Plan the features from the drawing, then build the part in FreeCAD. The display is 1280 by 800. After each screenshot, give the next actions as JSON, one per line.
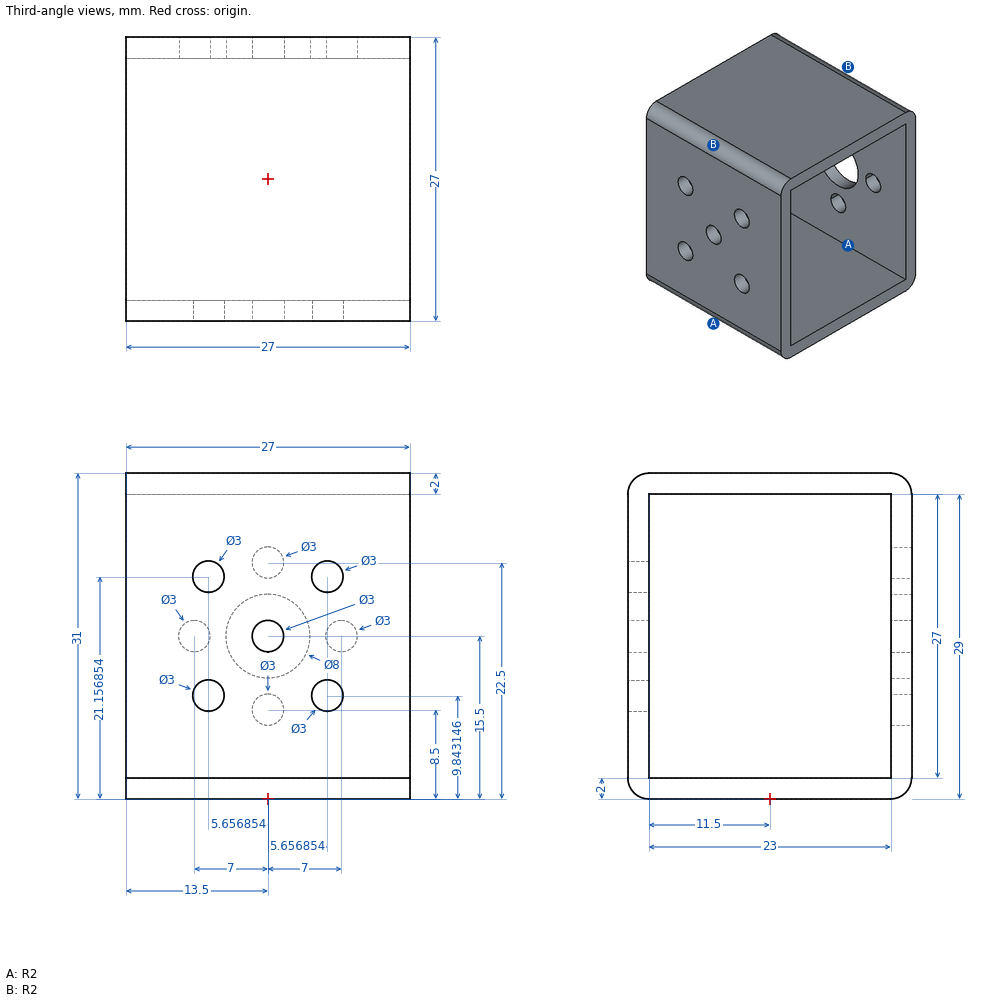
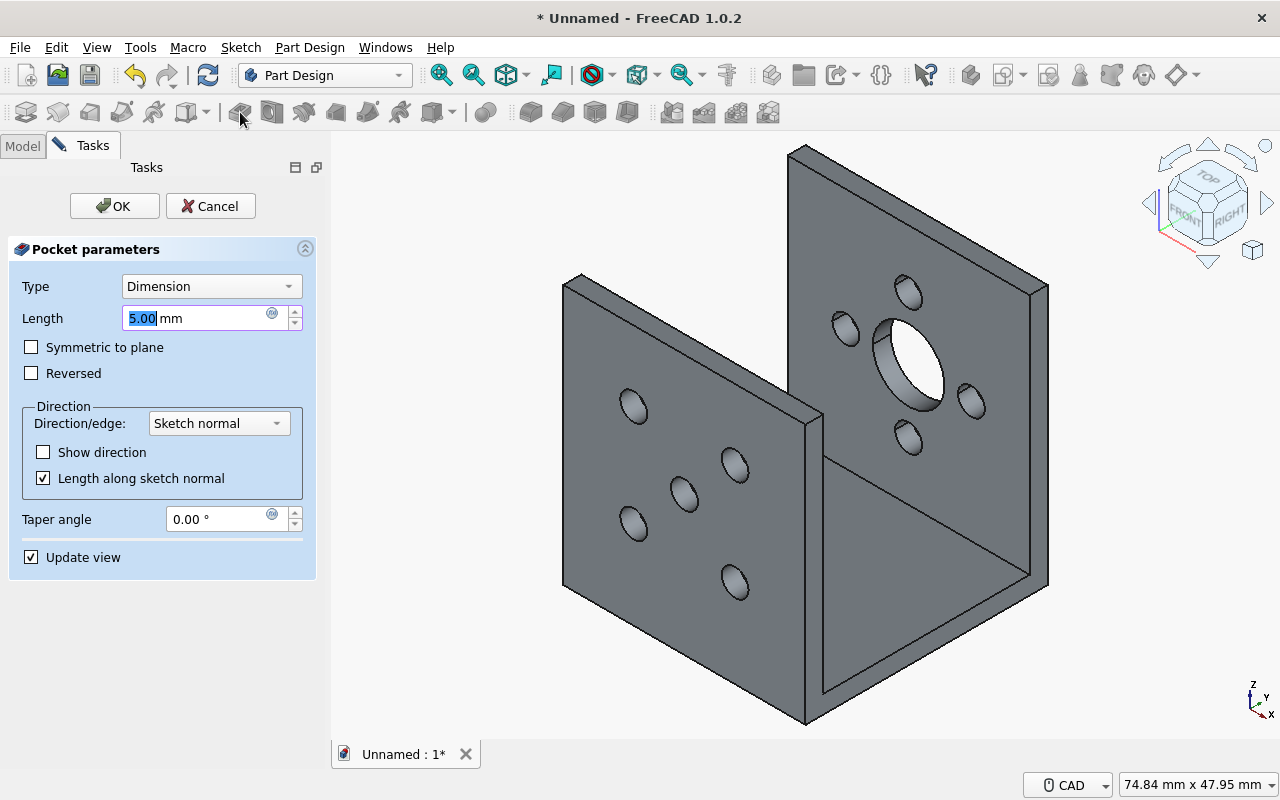
{"action": "left_click", "coordinate": [212, 286]}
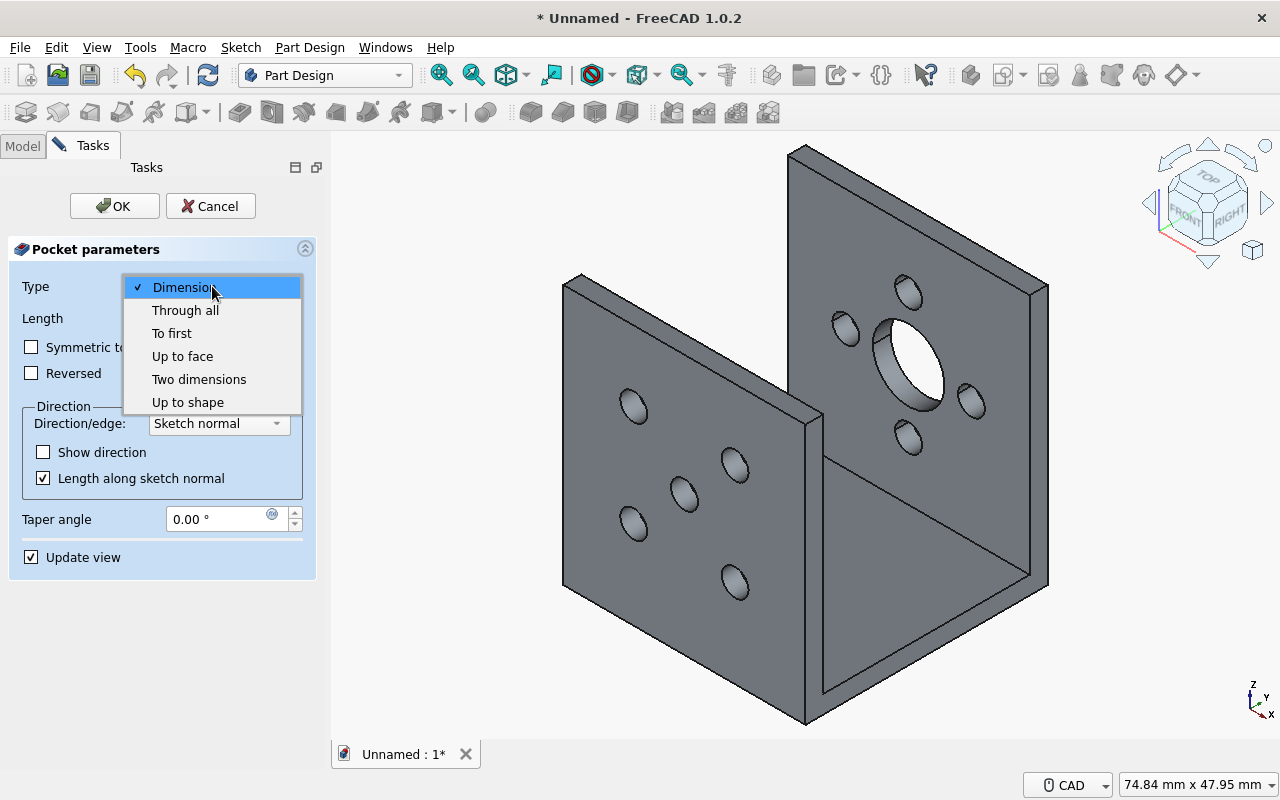
{"action": "left_click", "coordinate": [212, 334]}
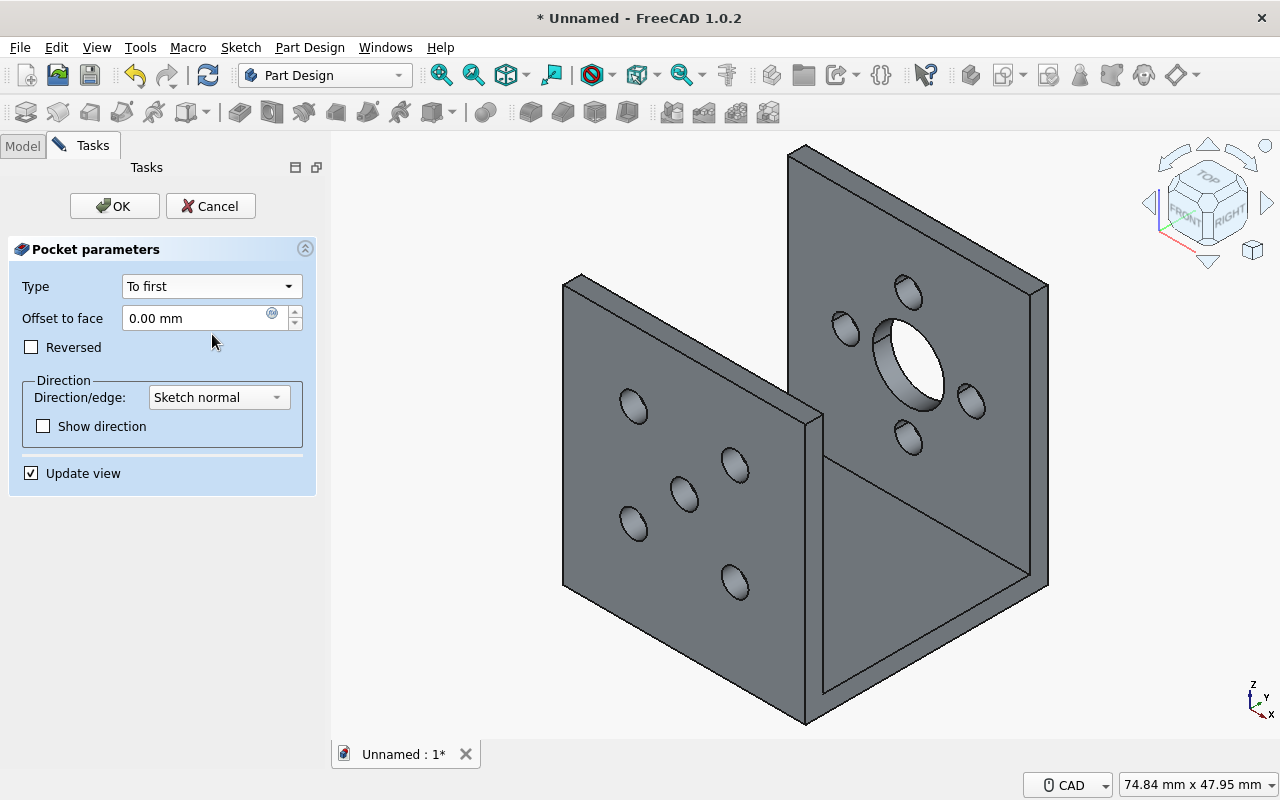
{"action": "left_click", "coordinate": [115, 206]}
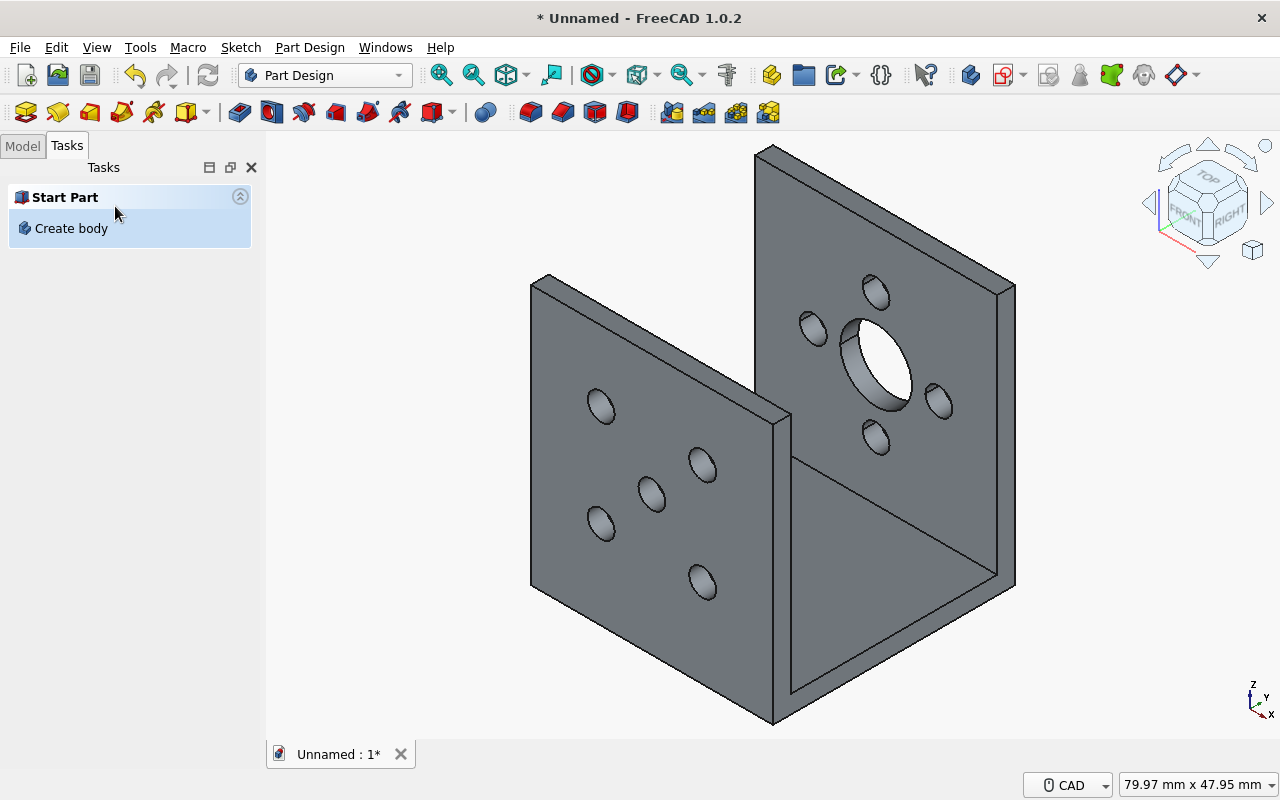
{"action": "key", "text": "2"}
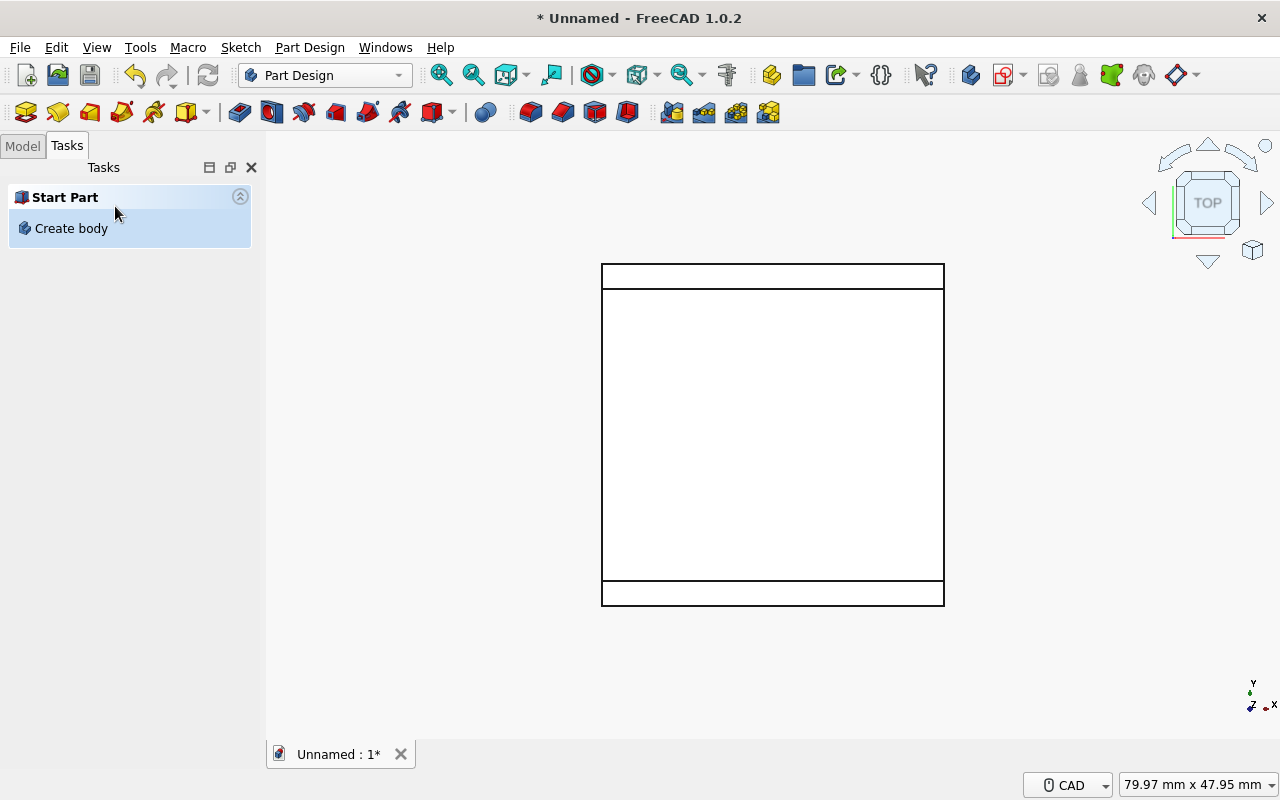
{"action": "key", "text": "0"}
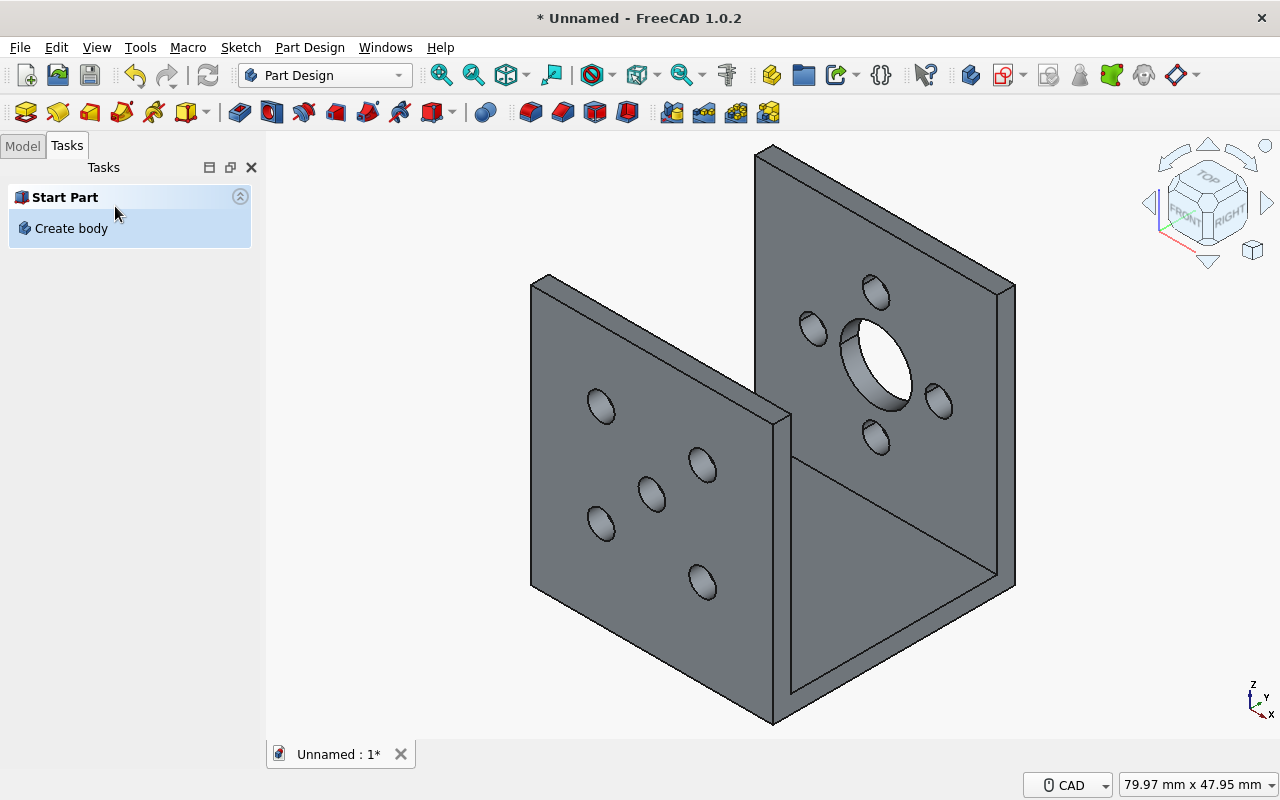
{"action": "key", "text": "1"}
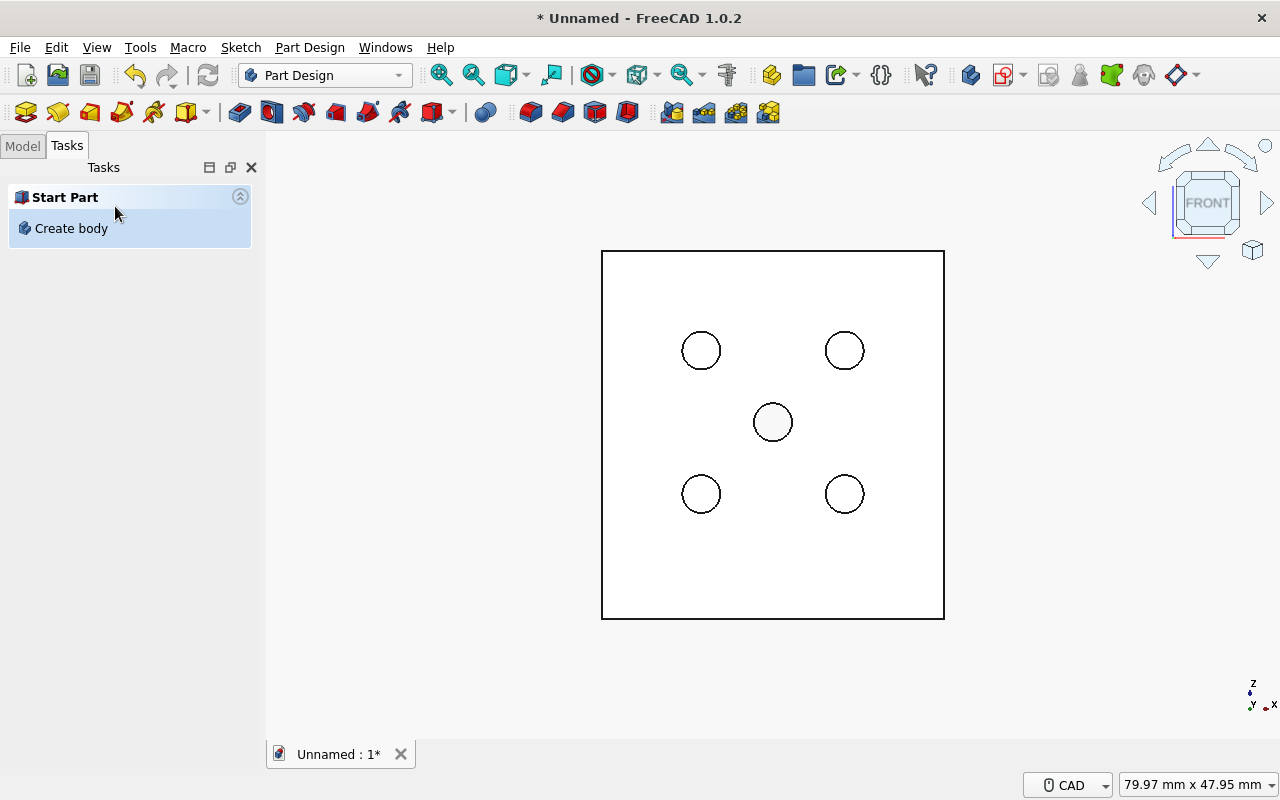
{"action": "left_click", "coordinate": [773, 618]}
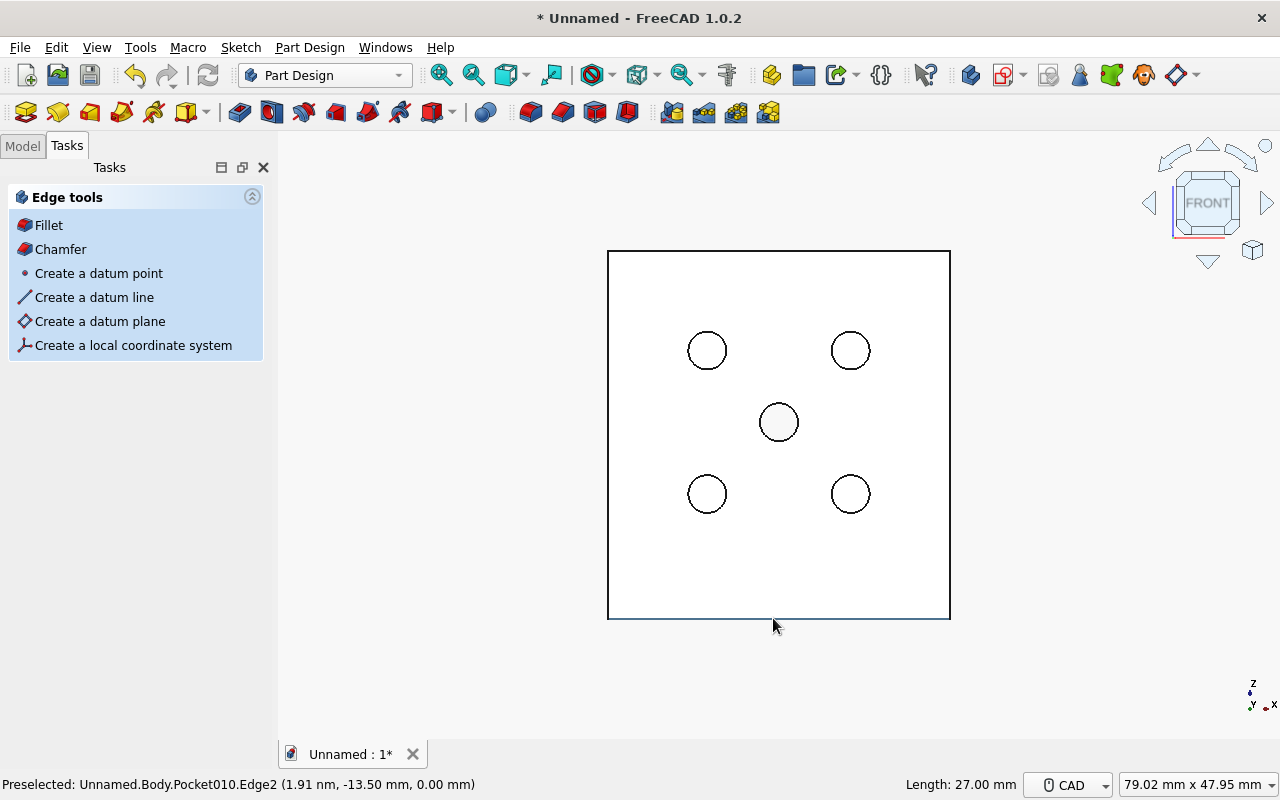
{"action": "key", "text": "3"}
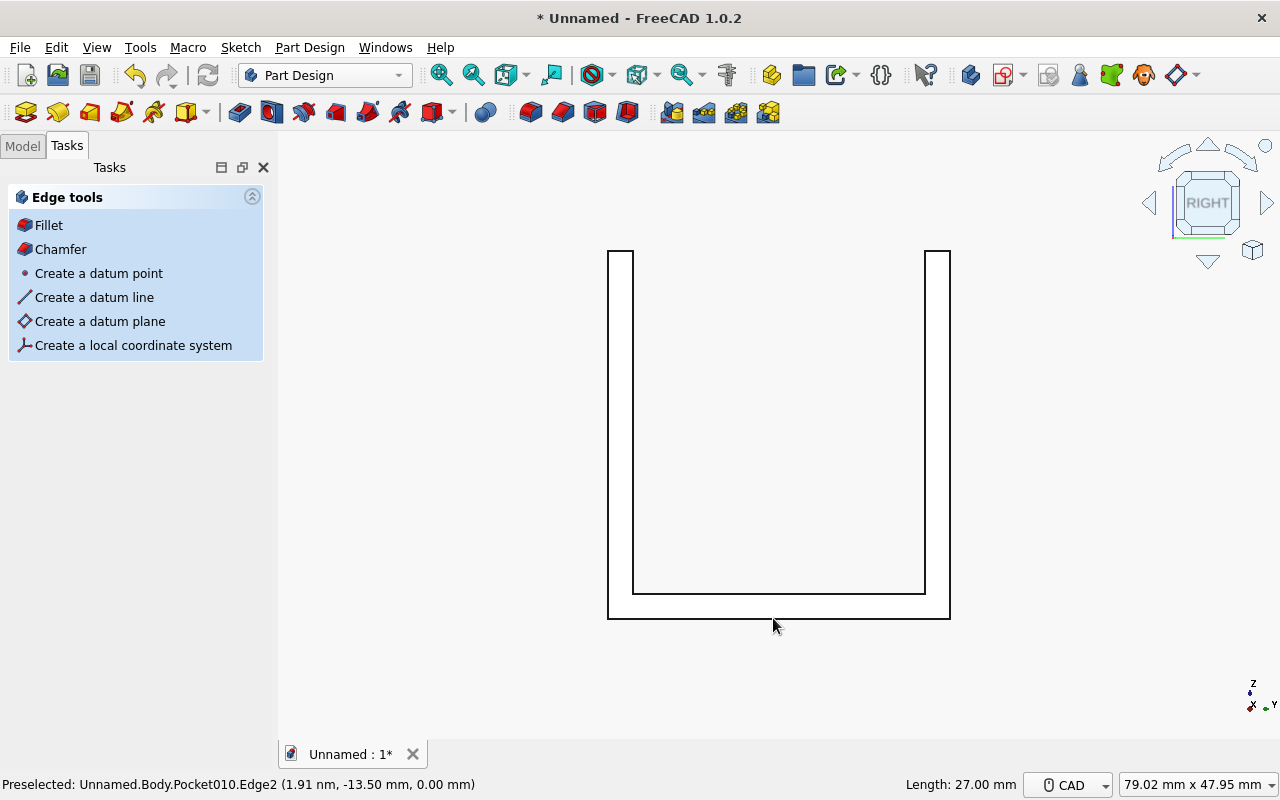
{"action": "key", "text": "5"}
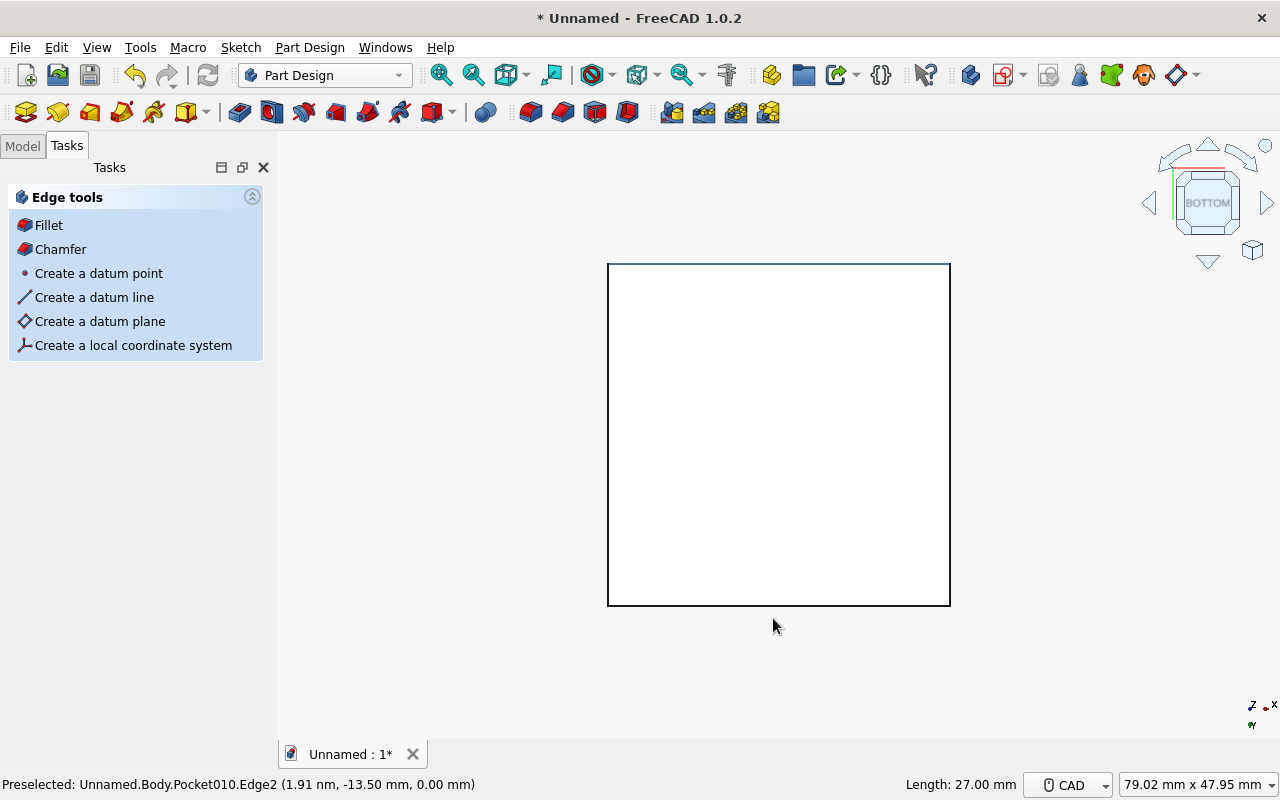
{"action": "left_click", "coordinate": [779, 605], "text": "ctrl"}